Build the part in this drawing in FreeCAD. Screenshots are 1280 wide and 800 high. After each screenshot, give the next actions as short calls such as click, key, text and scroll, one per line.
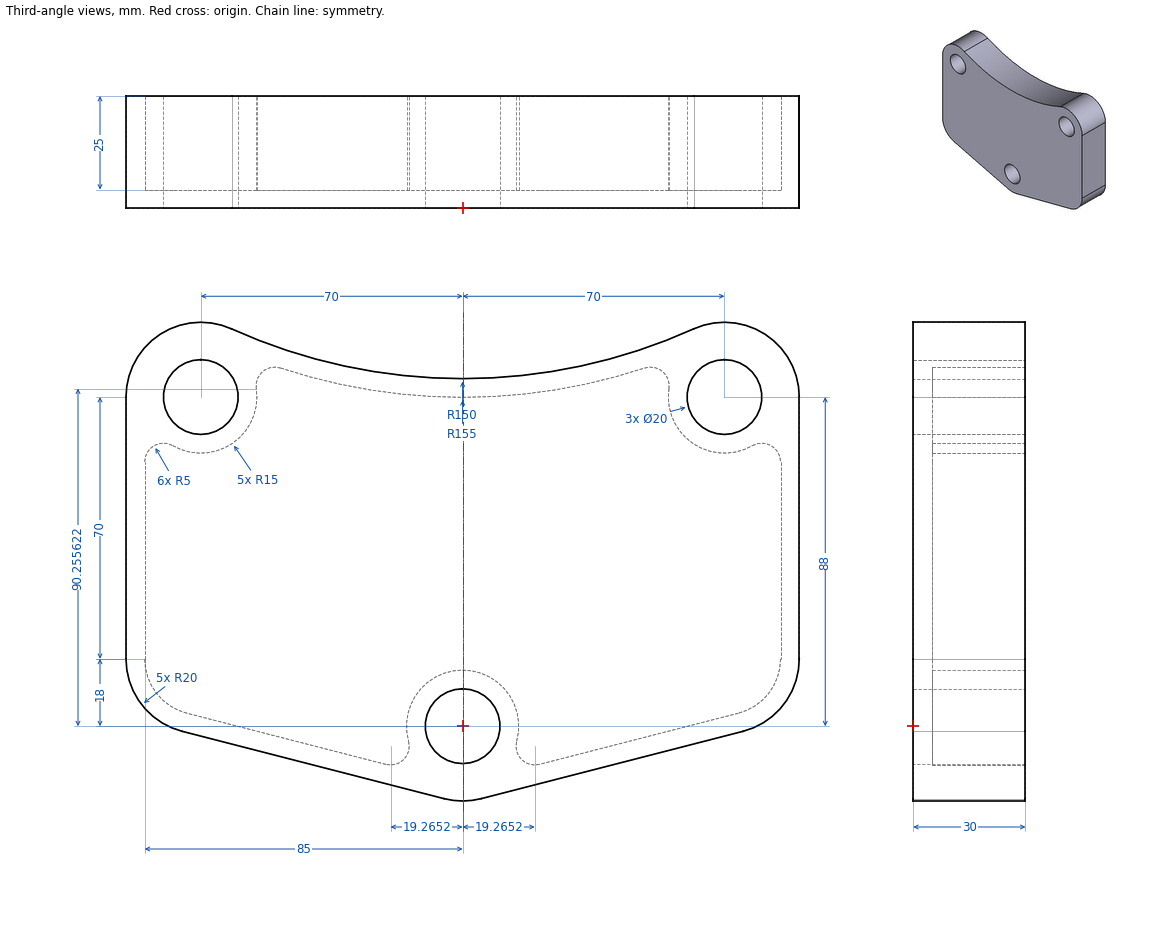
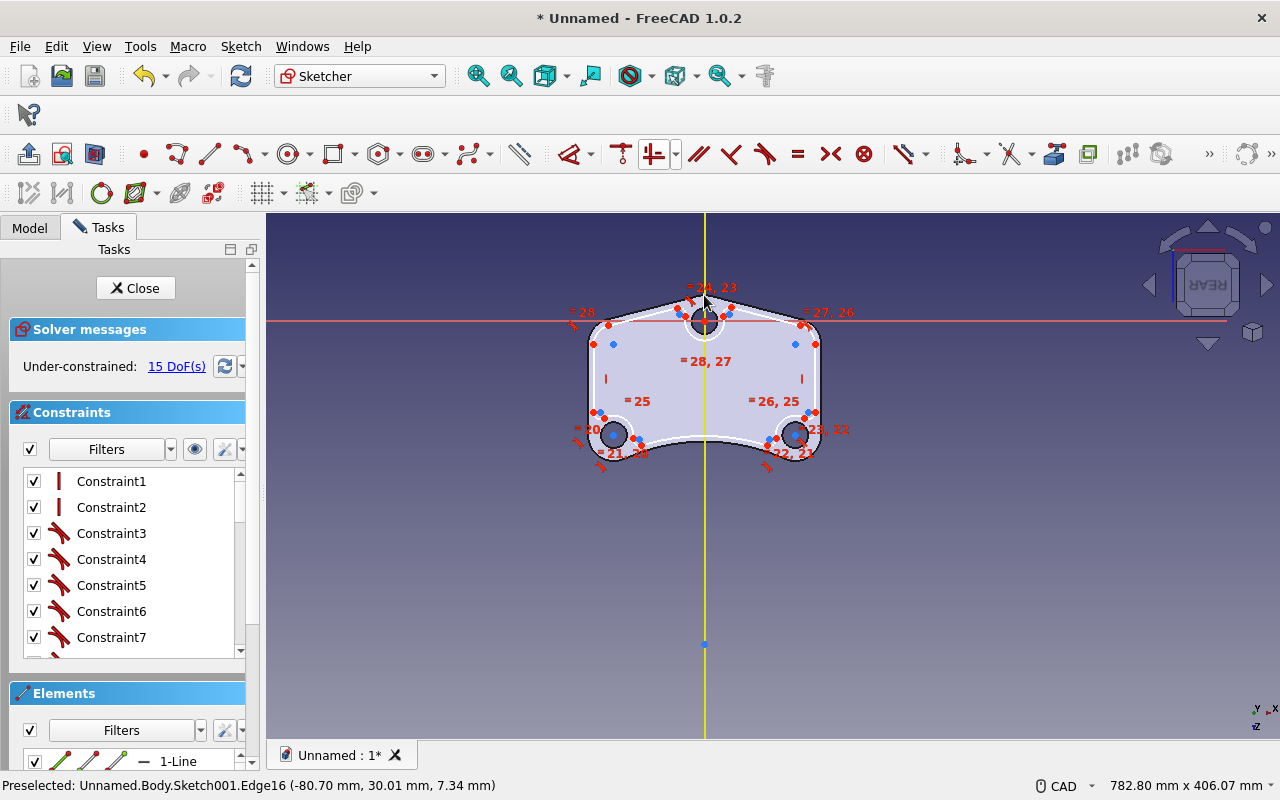
click(704, 644)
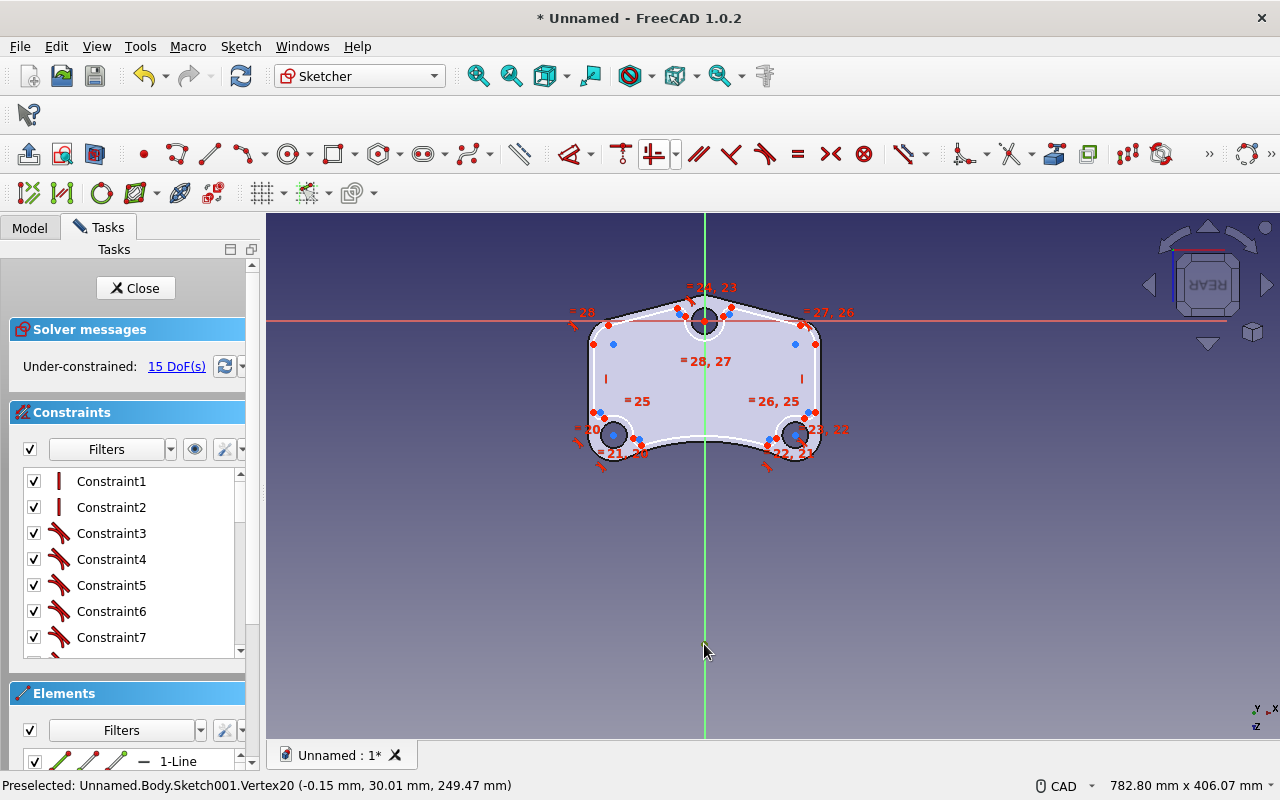
click(705, 677)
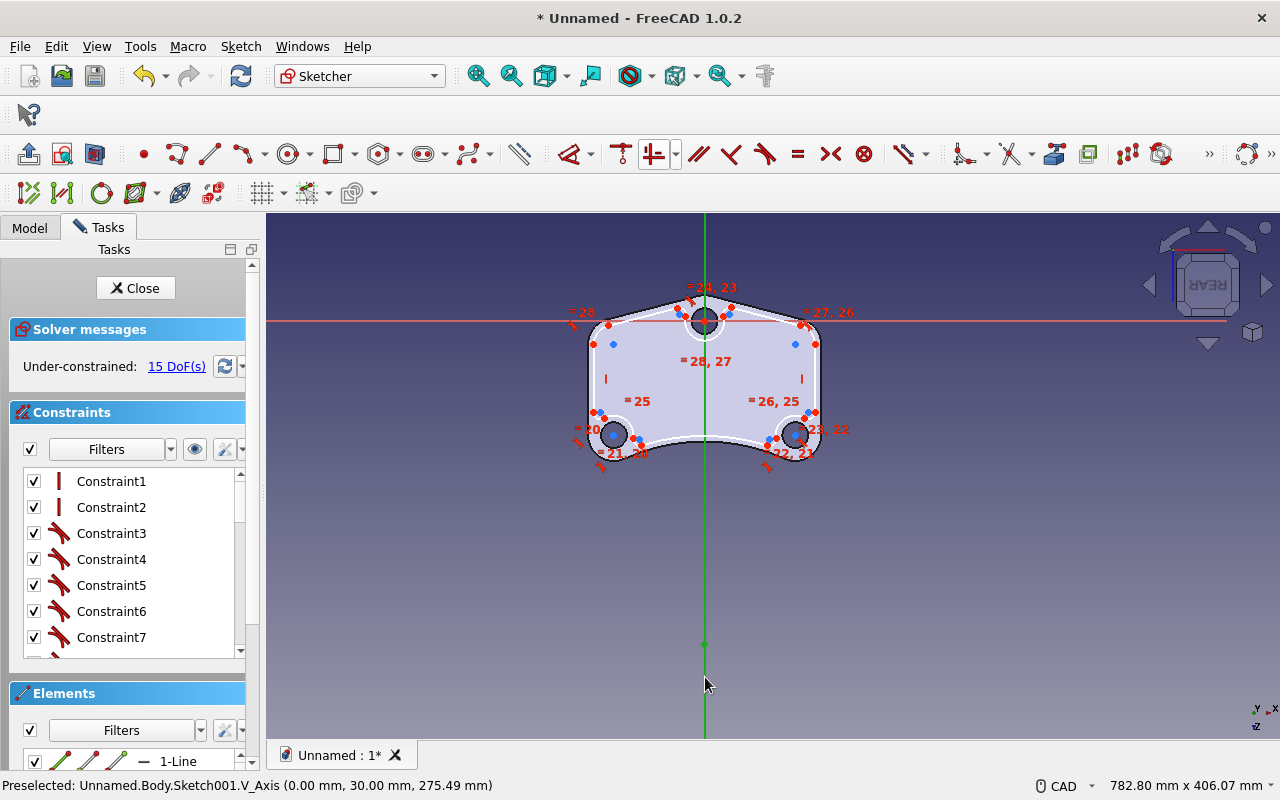
click(621, 154)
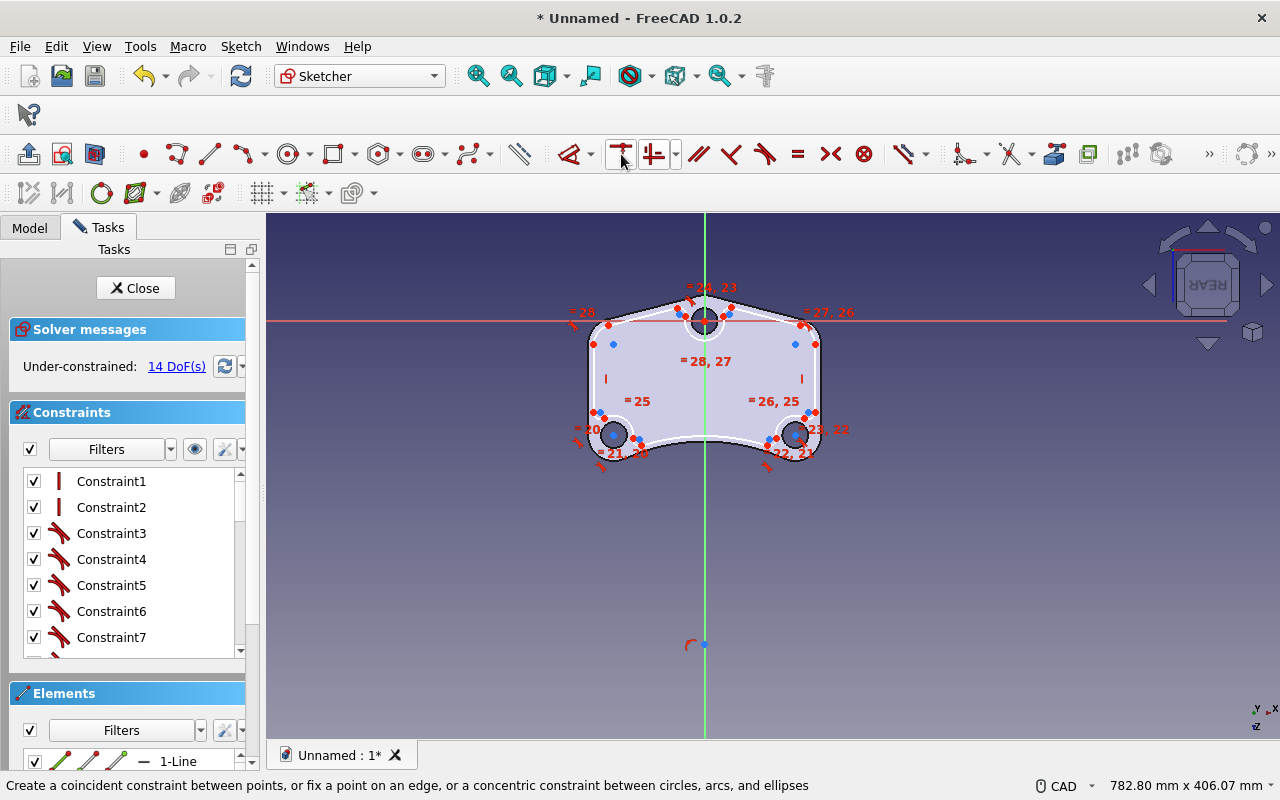
click(614, 435)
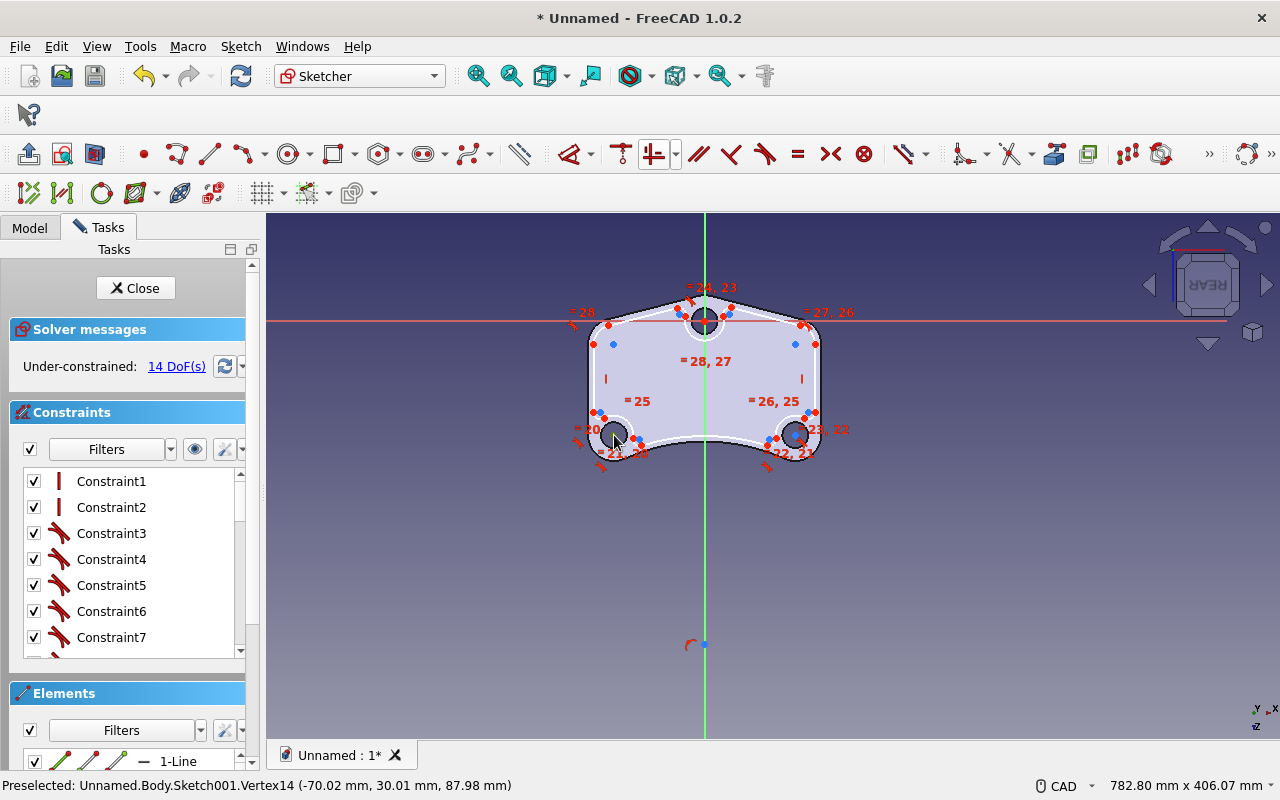
click(795, 435)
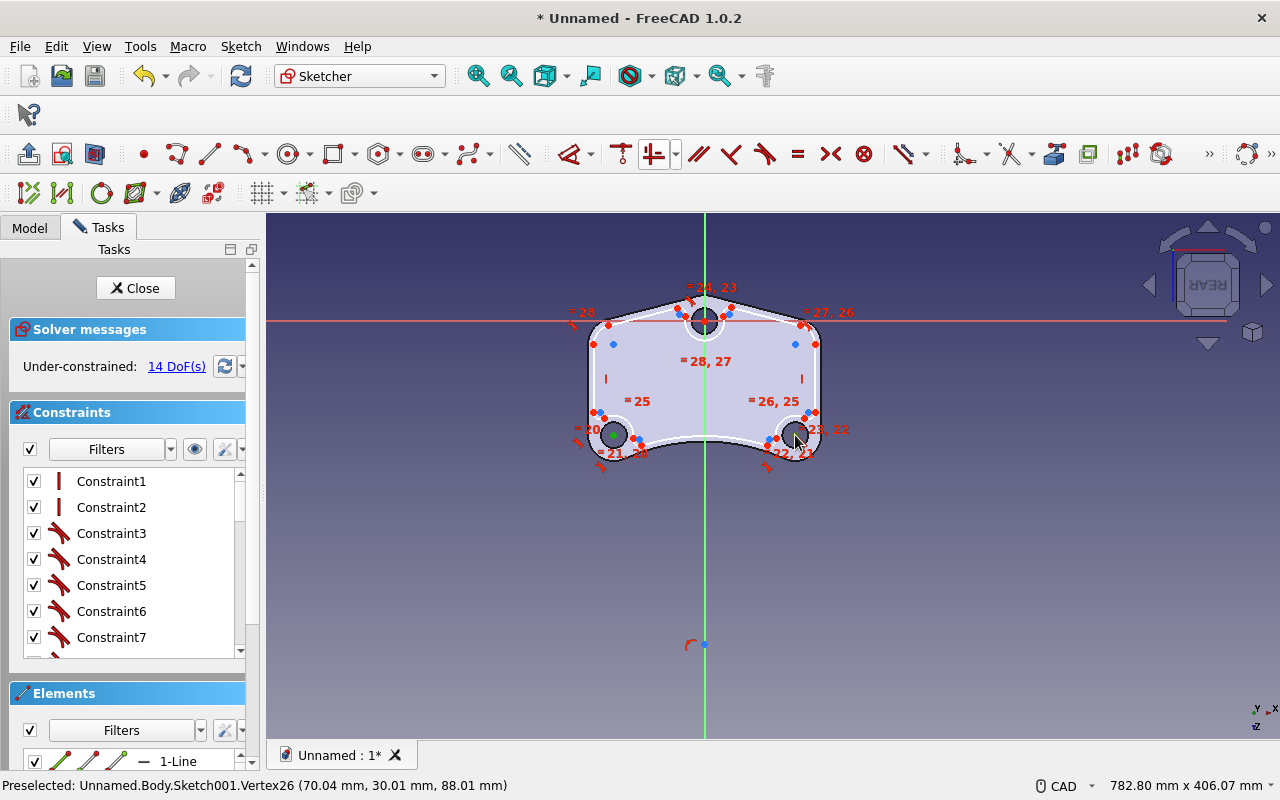
click(705, 677)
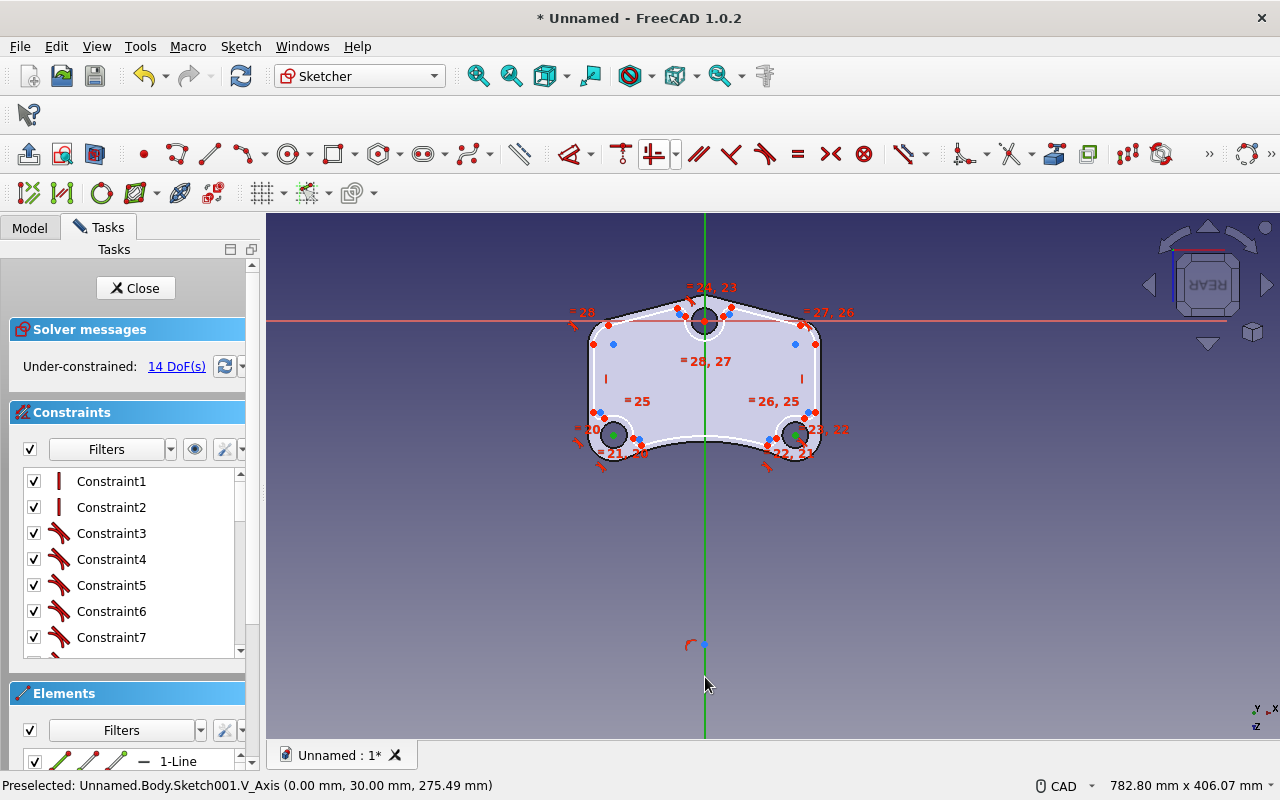
click(831, 154)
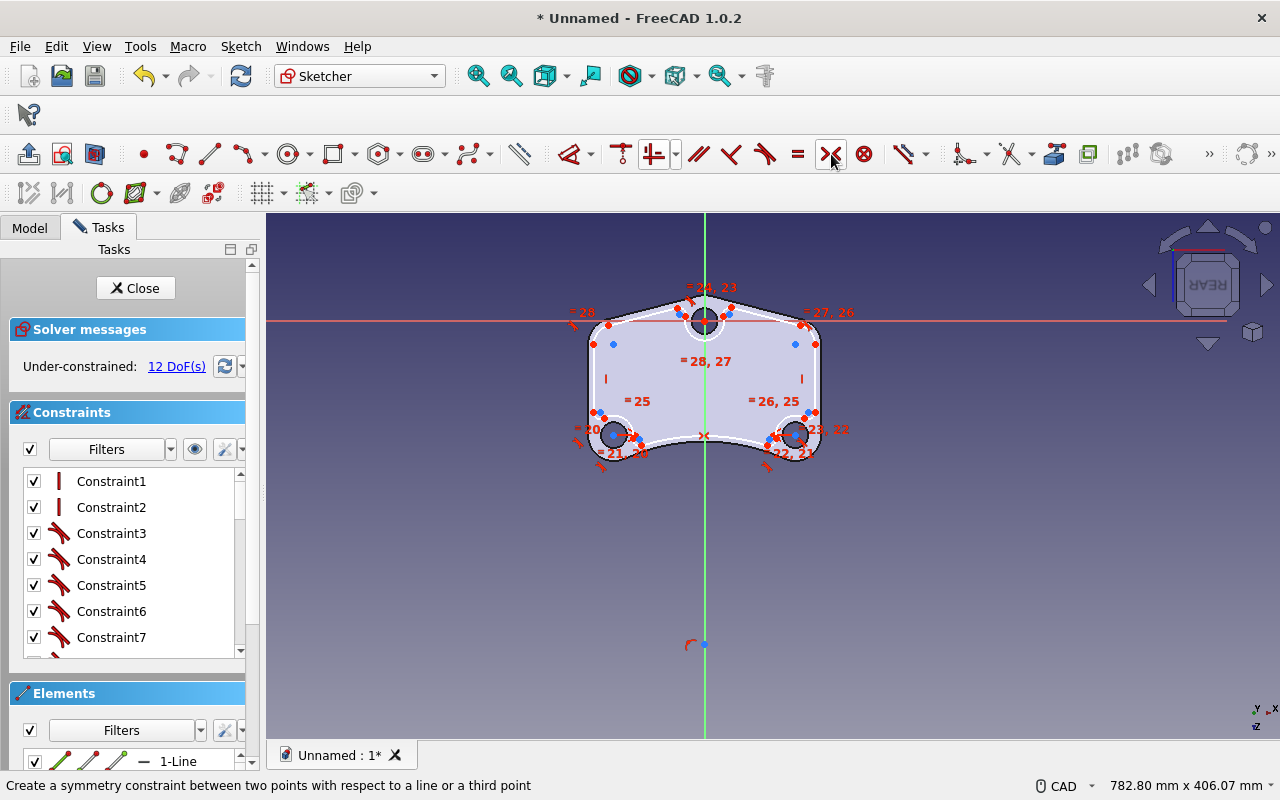
click(796, 345)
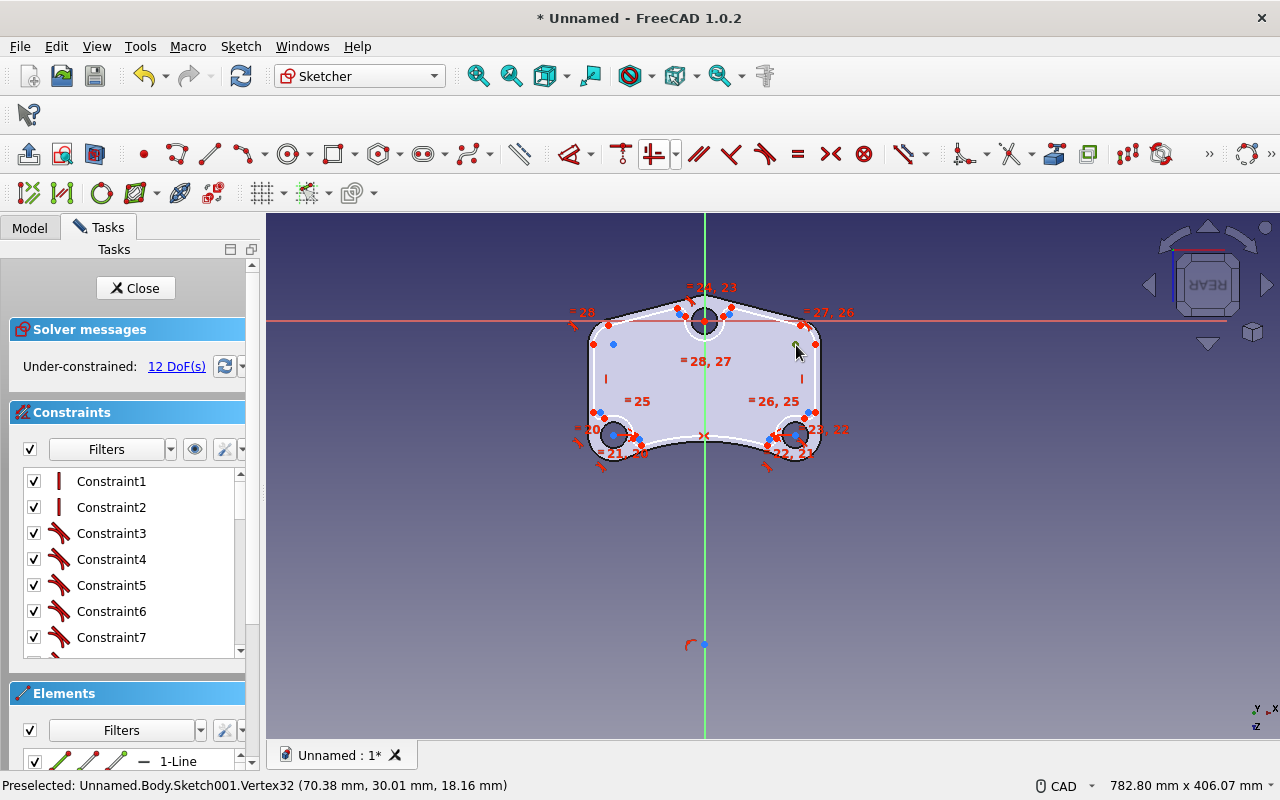
click(613, 345)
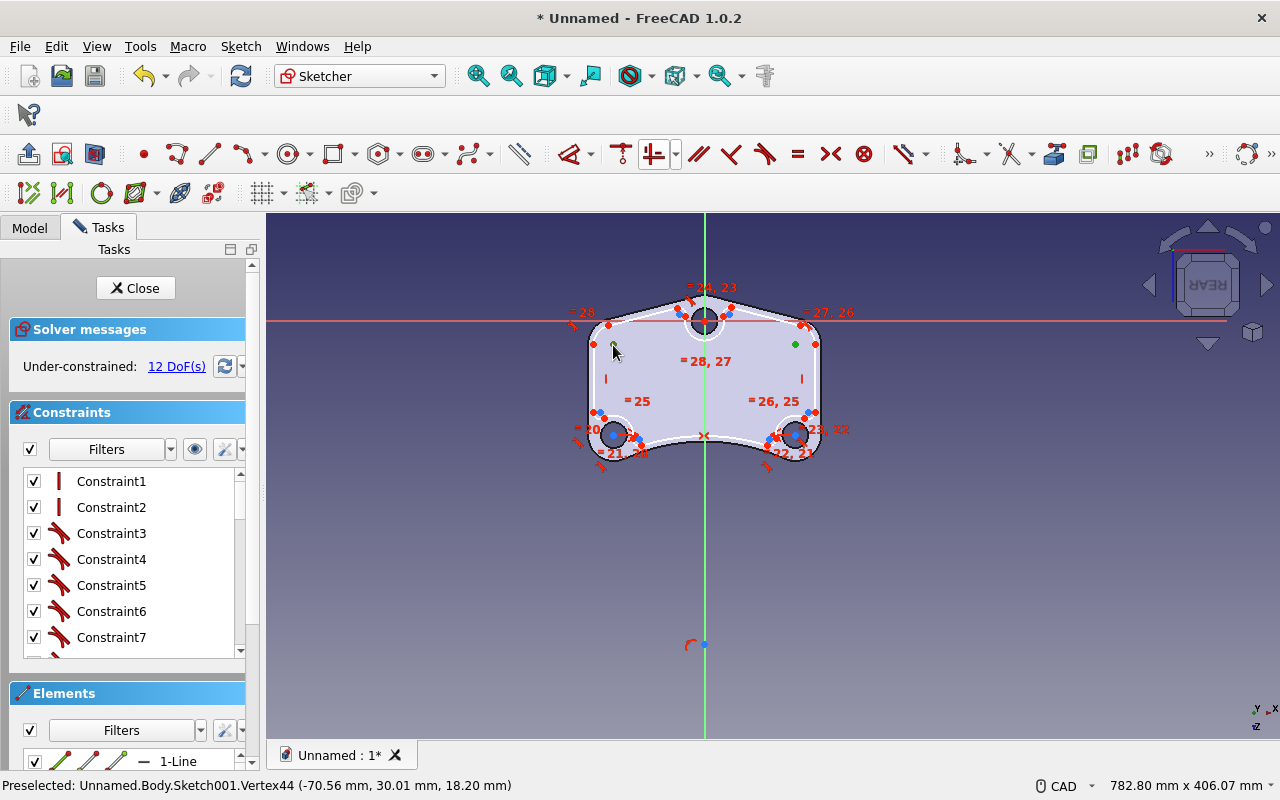
click(705, 677)